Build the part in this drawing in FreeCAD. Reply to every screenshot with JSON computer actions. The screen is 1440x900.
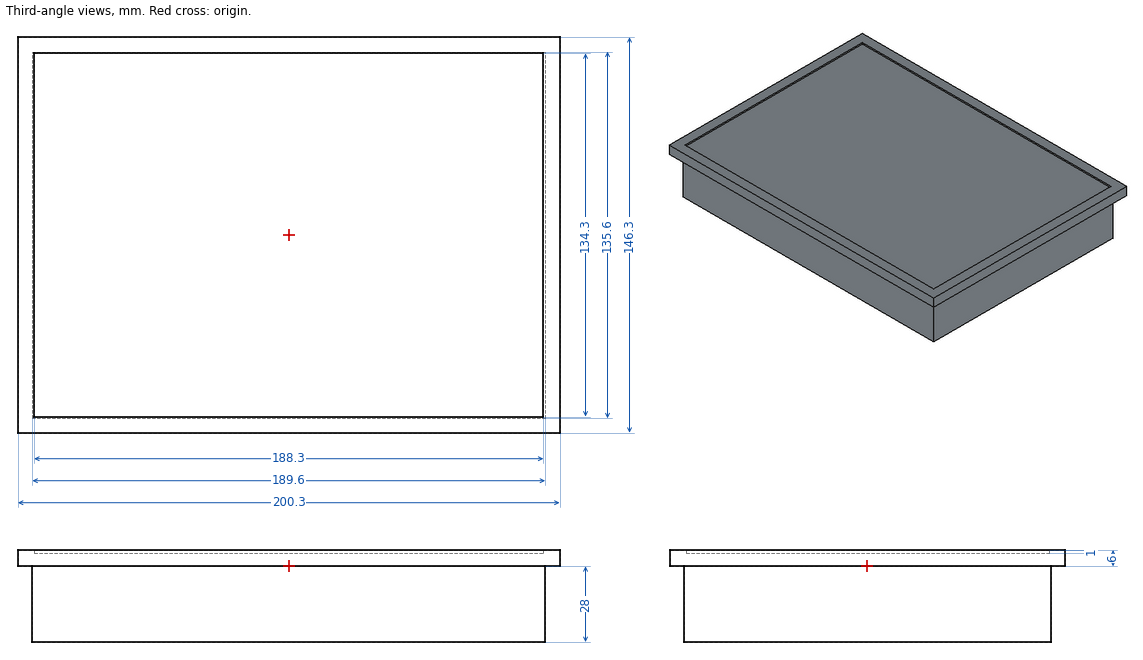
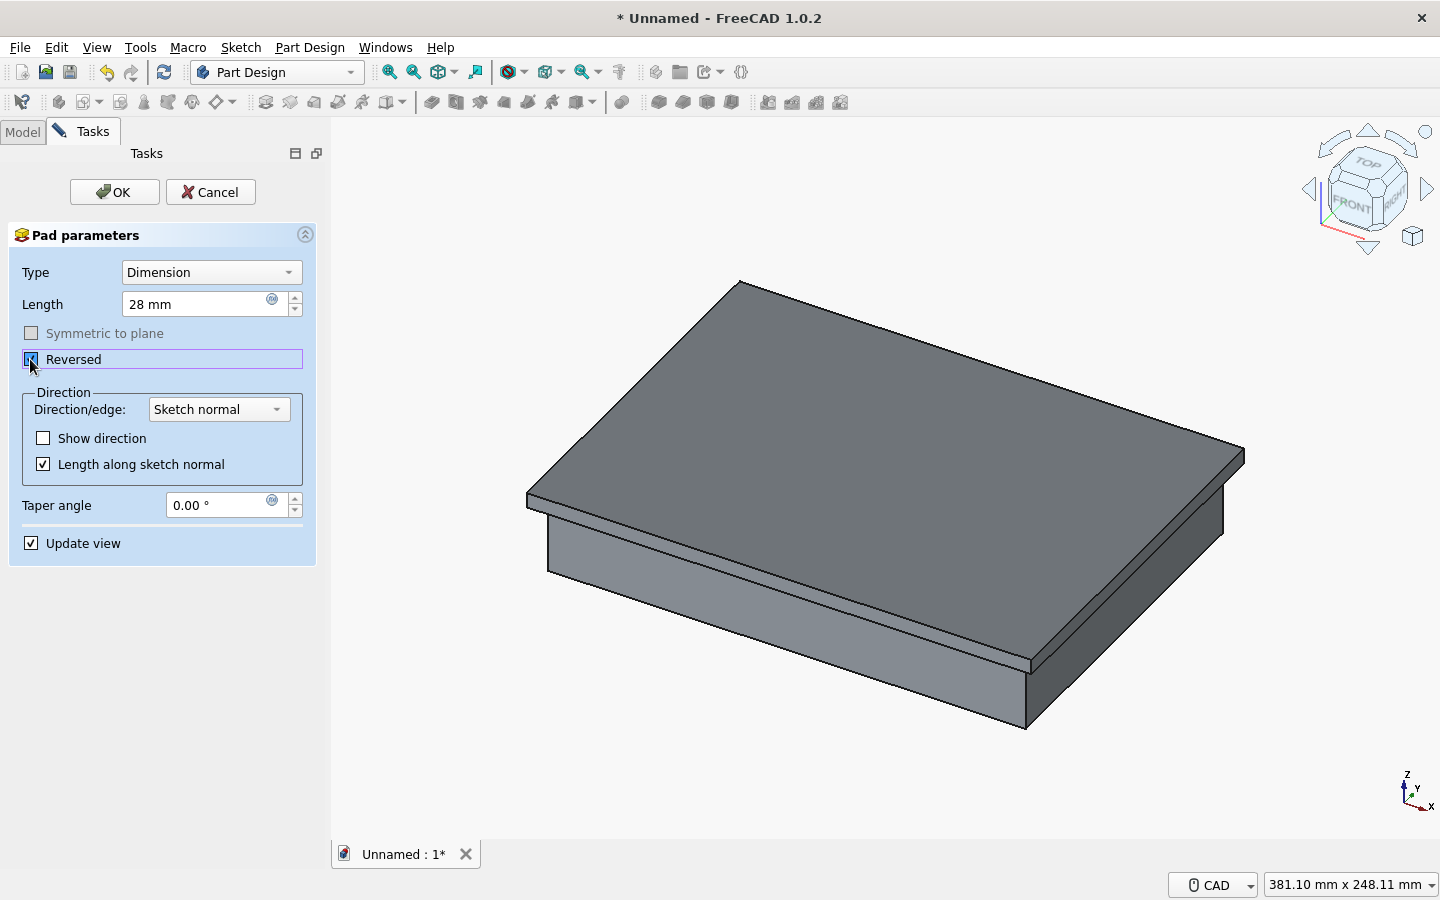
{"action": "left_click", "coordinate": [115, 192]}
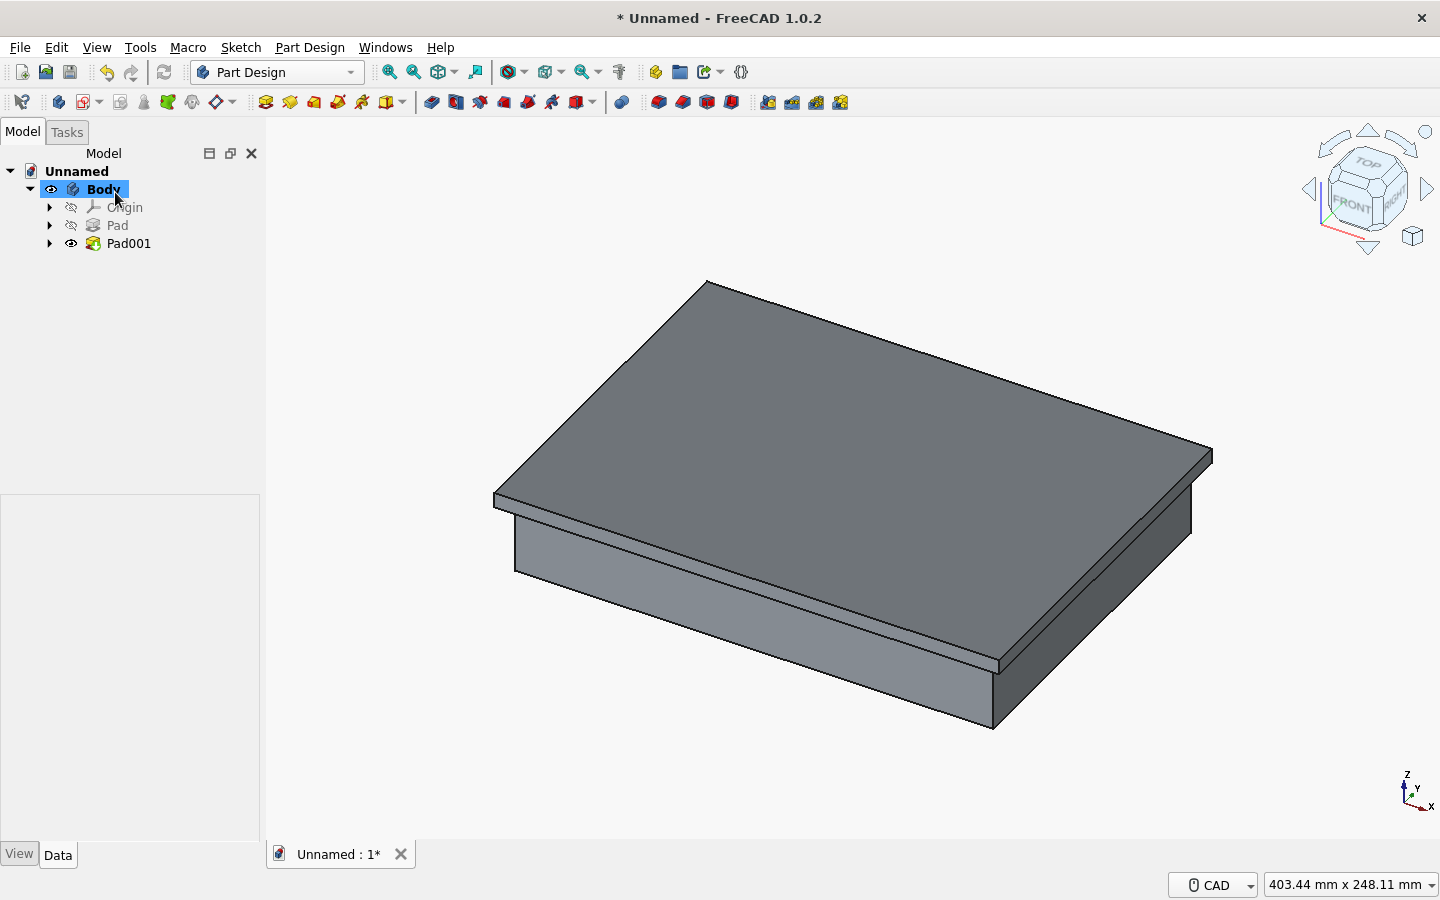
{"action": "left_click", "coordinate": [853, 470]}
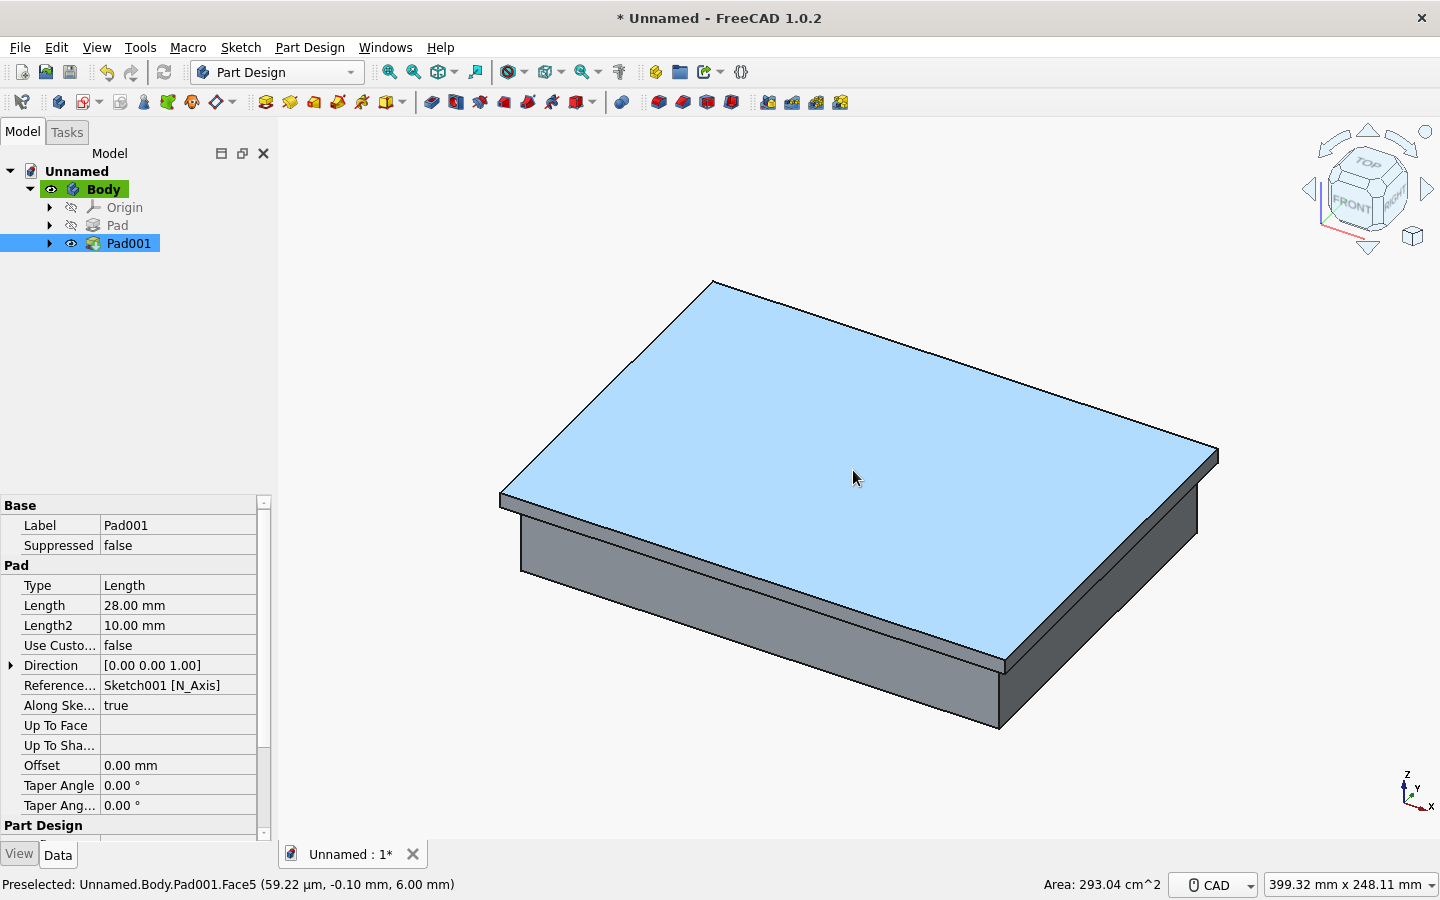
{"action": "left_click", "coordinate": [84, 102]}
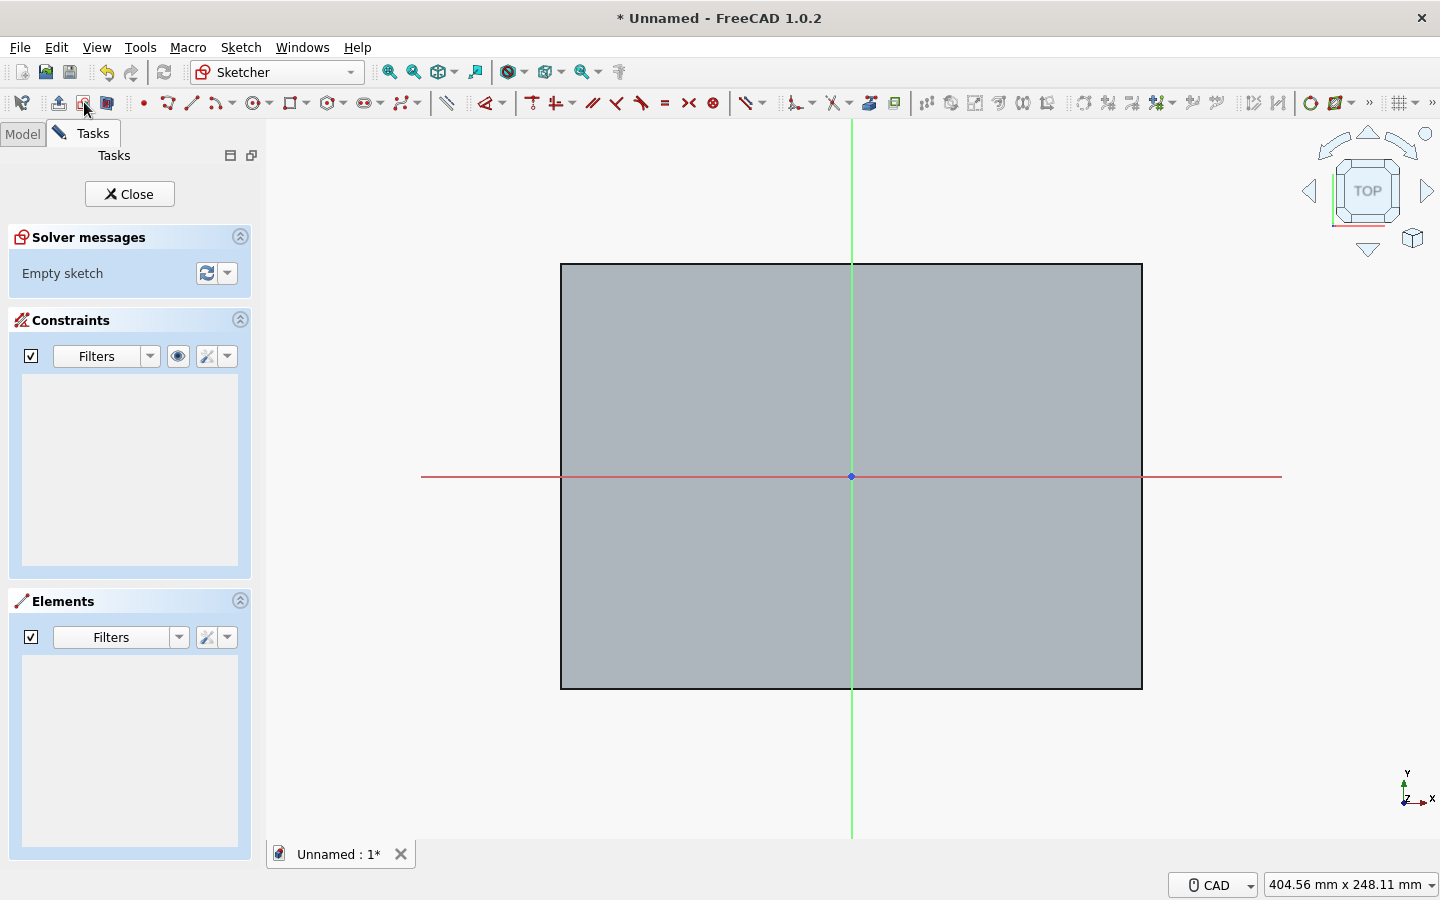
{"action": "key", "text": "g v"}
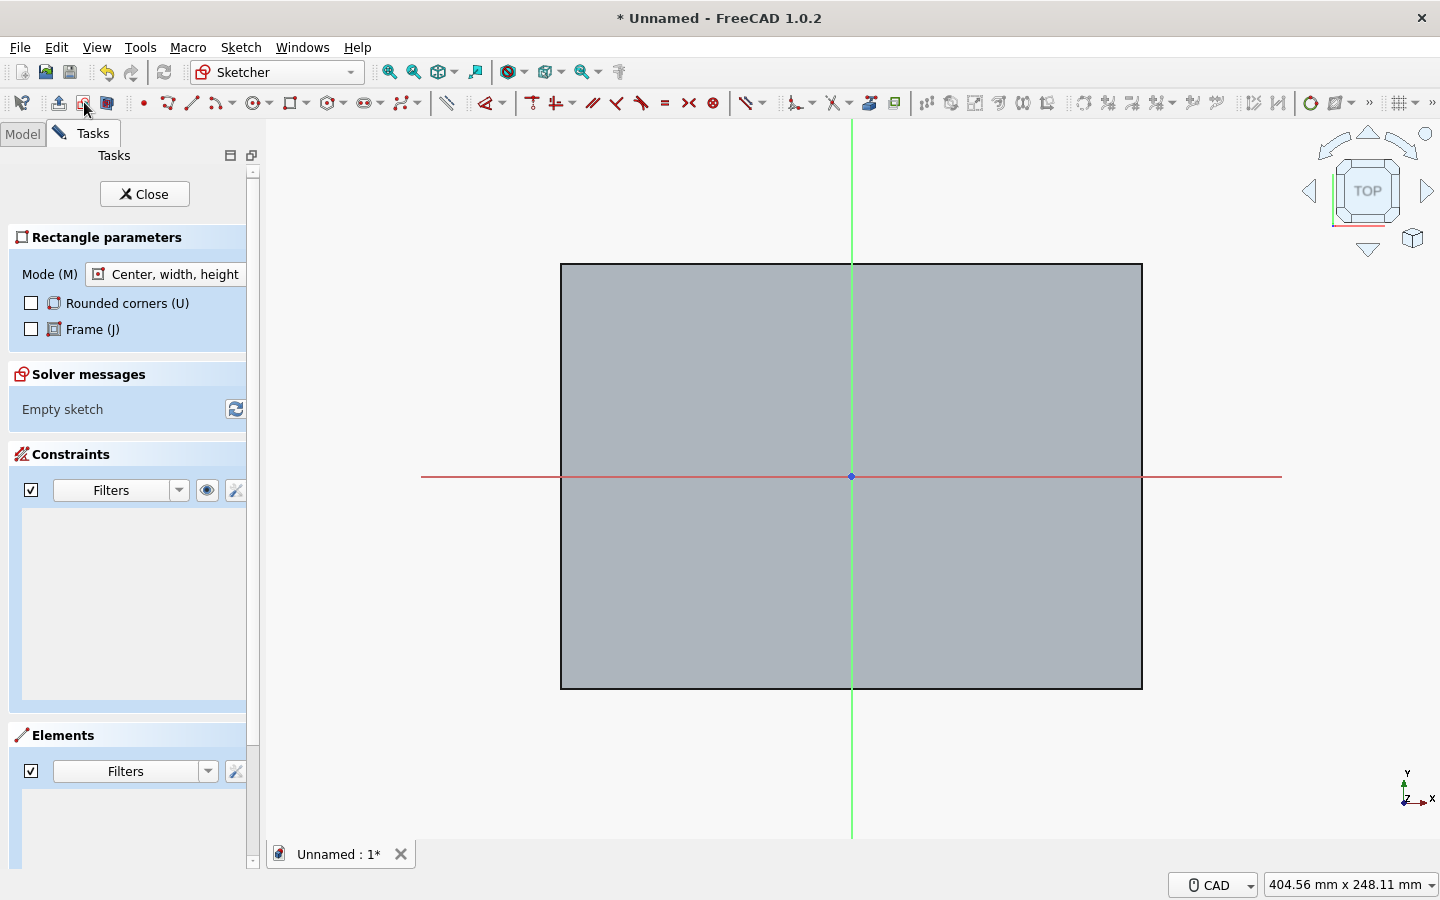
{"action": "left_click", "coordinate": [852, 477]}
{"action": "left_click", "coordinate": [1125, 282]}
{"action": "key", "text": "Escape"}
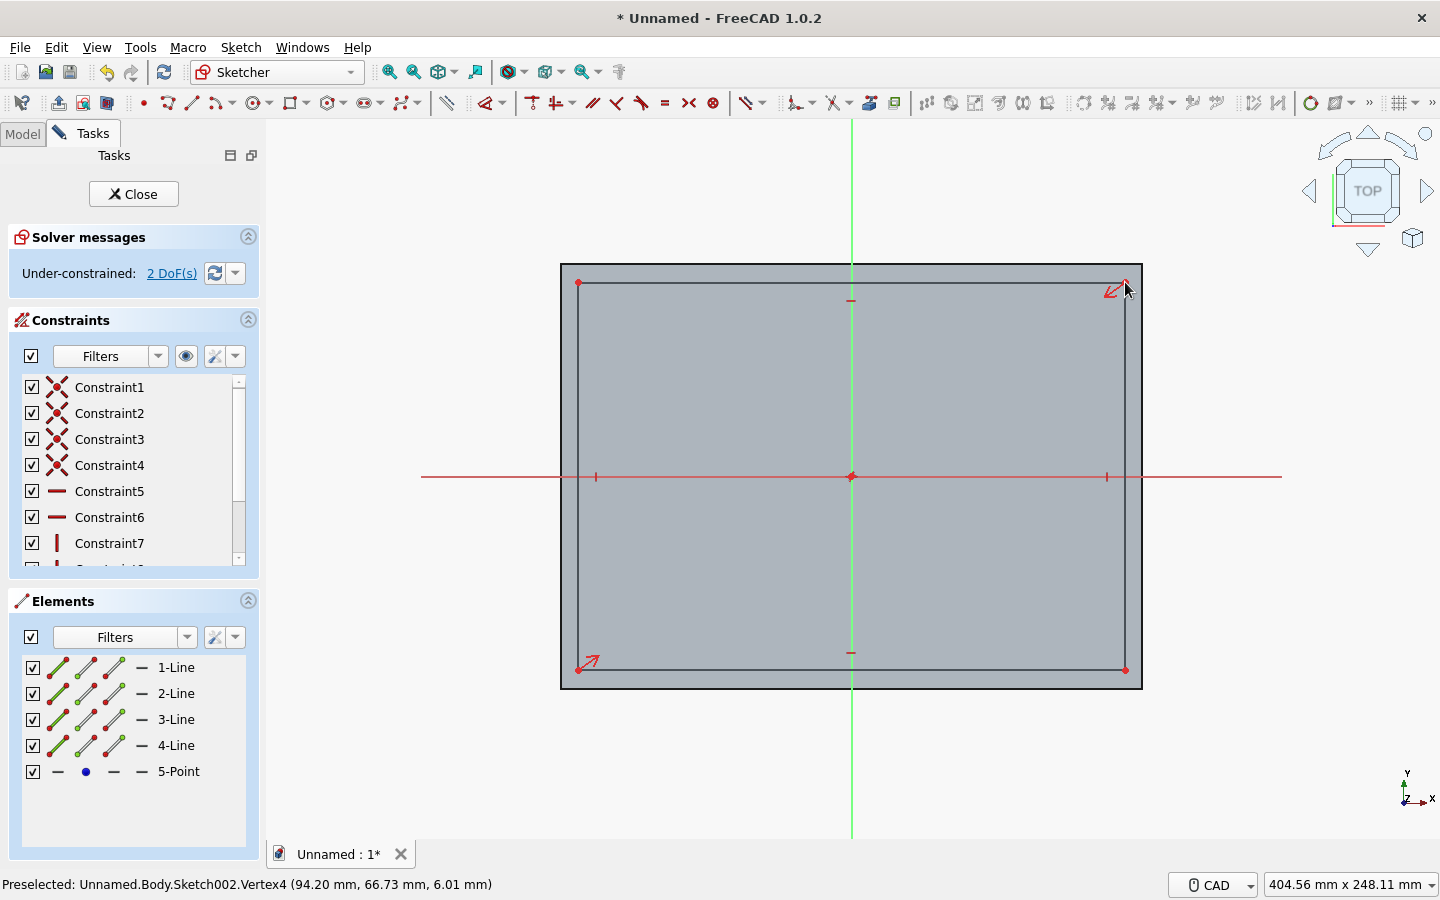
{"action": "left_click", "coordinate": [486, 104]}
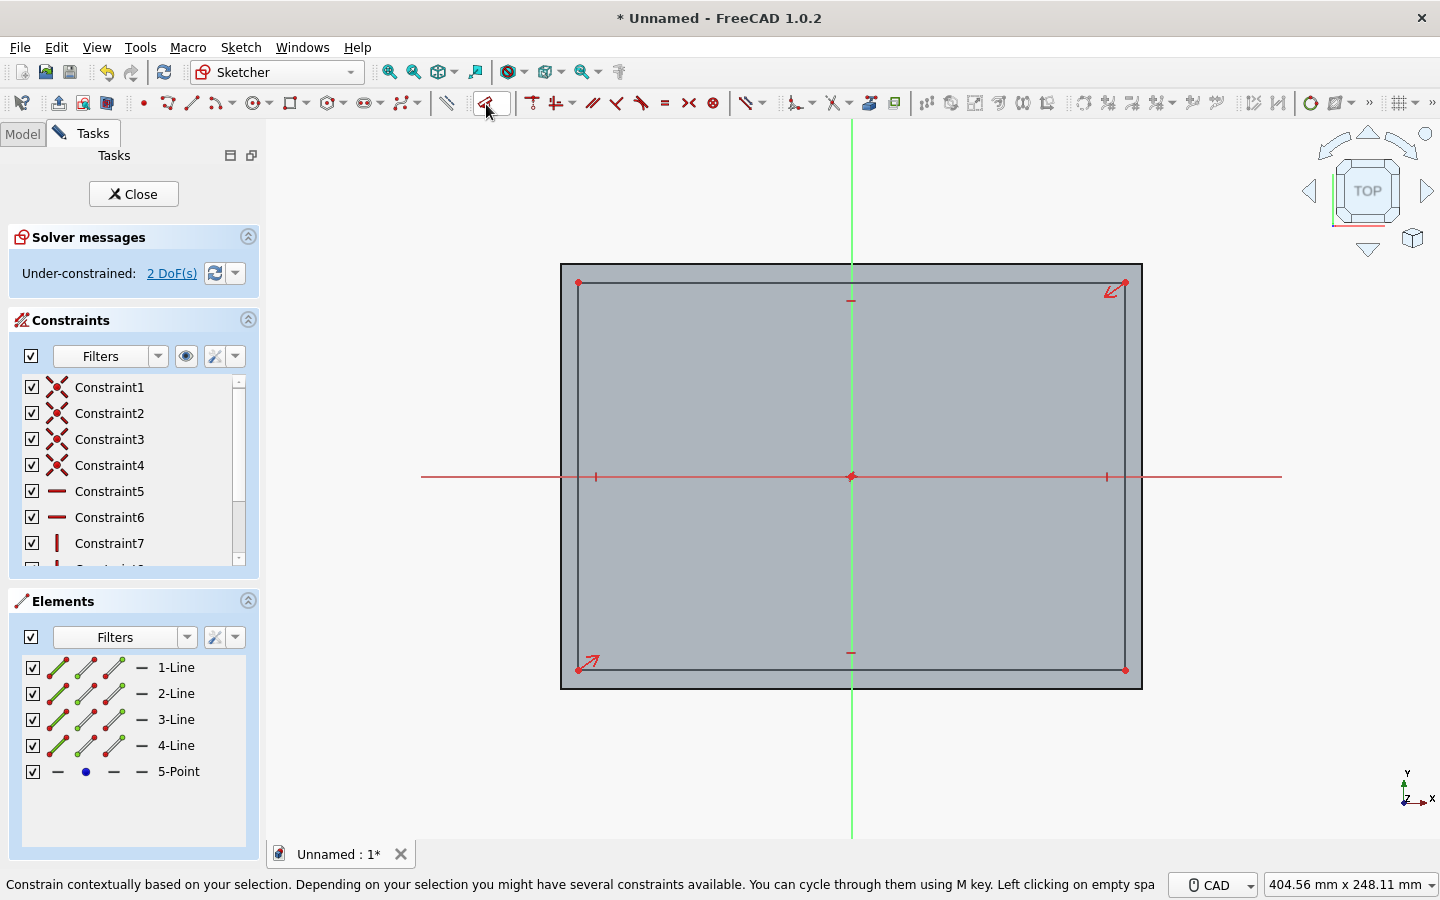
{"action": "left_click", "coordinate": [742, 670]}
{"action": "left_click", "coordinate": [726, 704]}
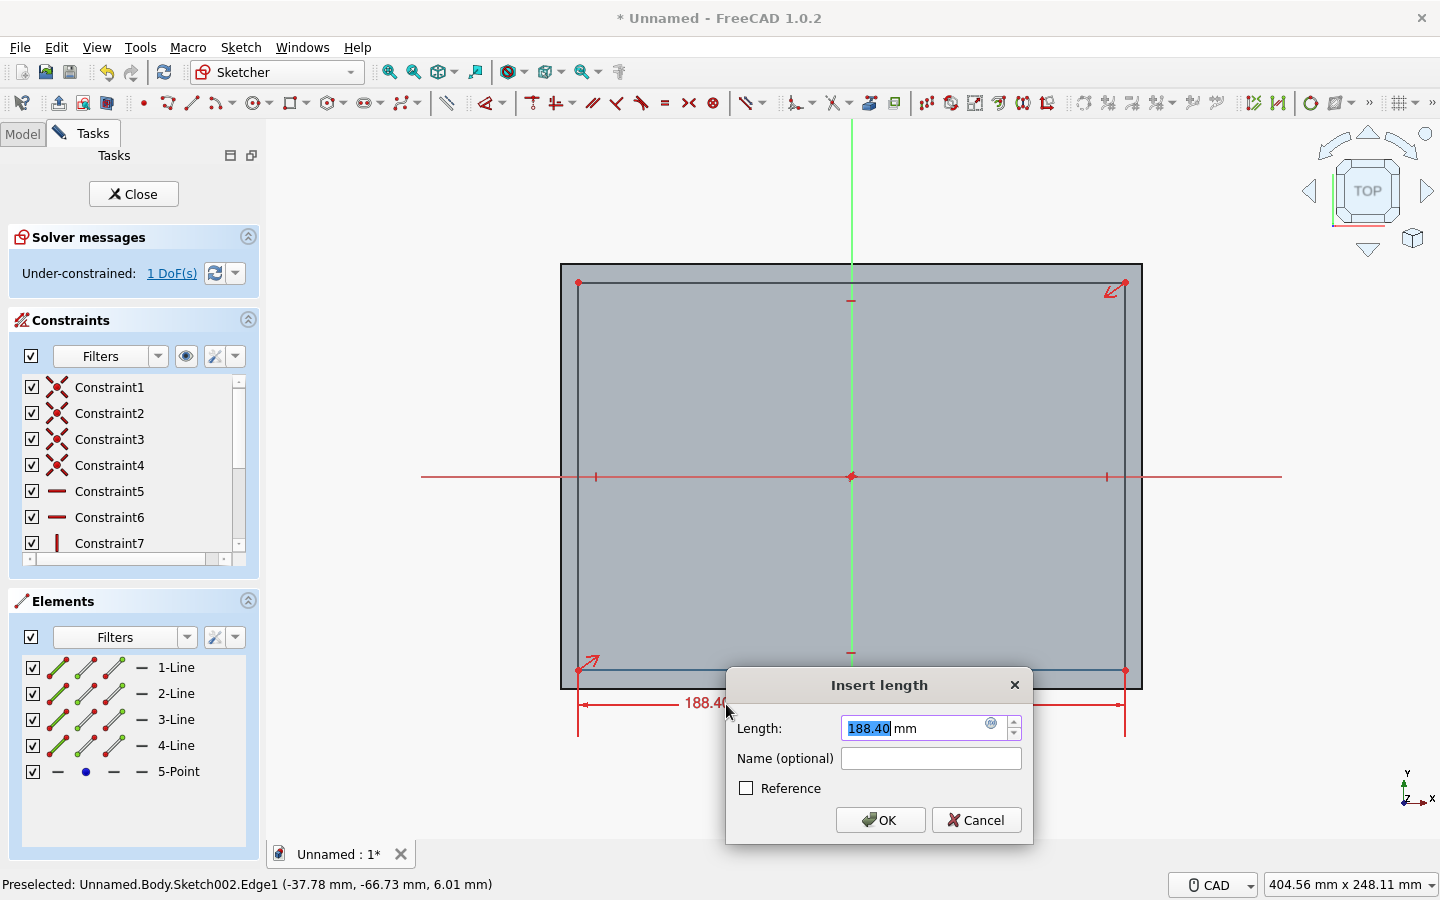
{"action": "type", "text": "188.3"}
{"action": "key", "text": "Return"}